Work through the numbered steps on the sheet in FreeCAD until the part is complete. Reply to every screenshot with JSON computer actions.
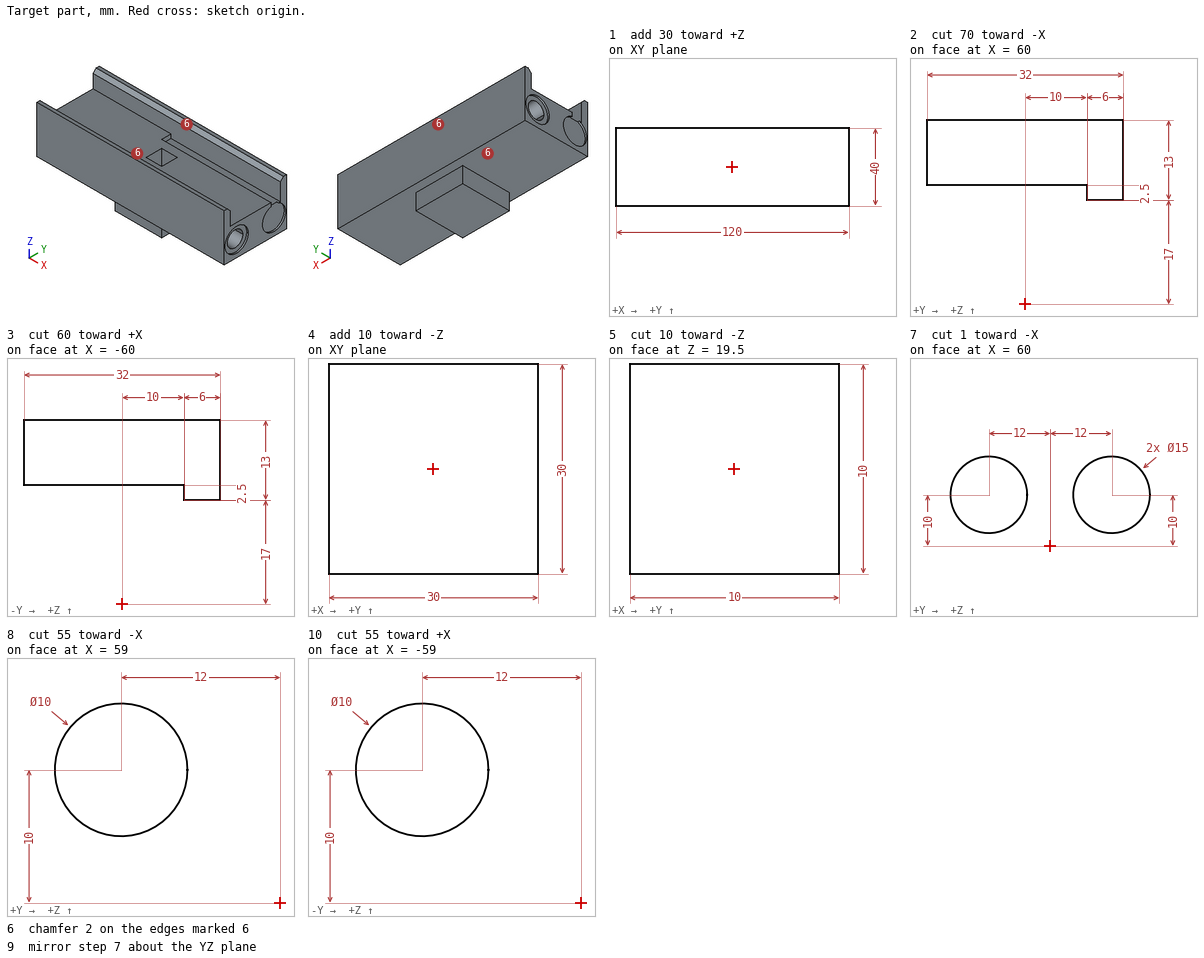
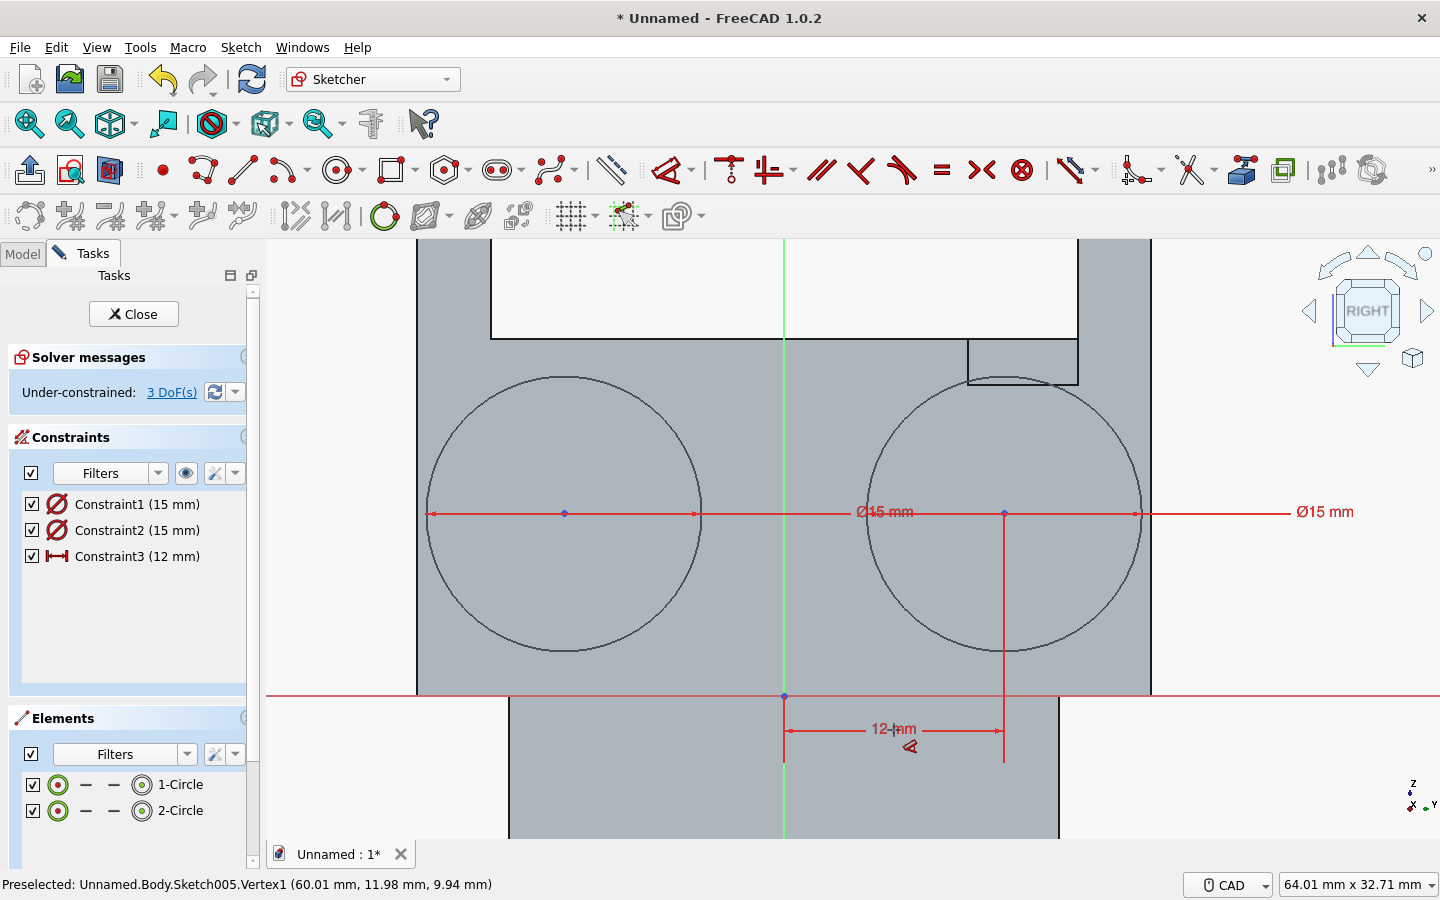
{"action": "left_click", "coordinate": [1004, 514]}
{"action": "left_click", "coordinate": [1038, 605]}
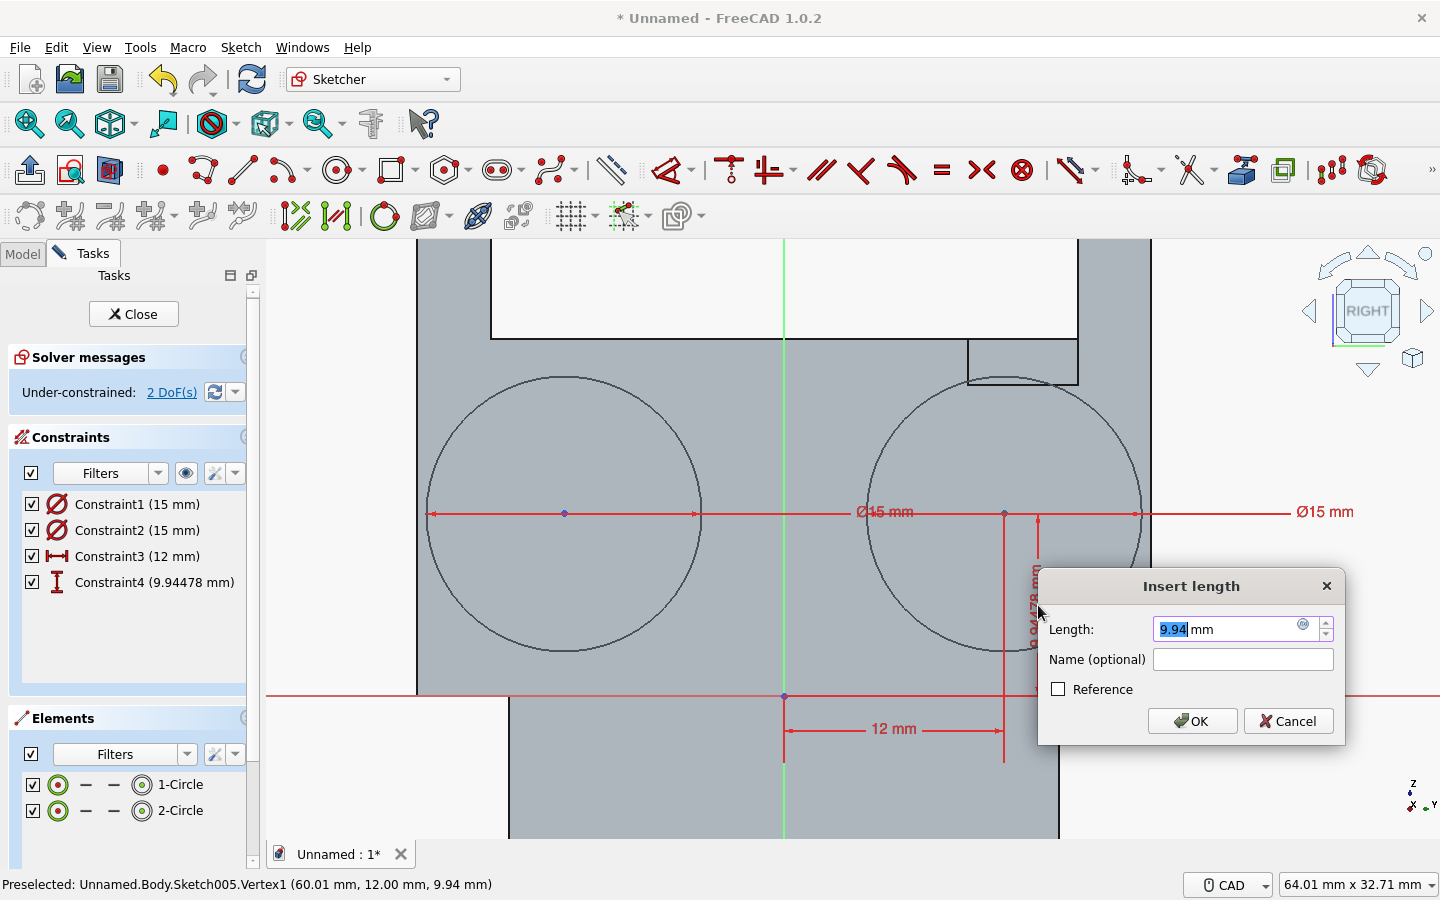
{"action": "type", "text": "10"}
{"action": "key", "text": "Return"}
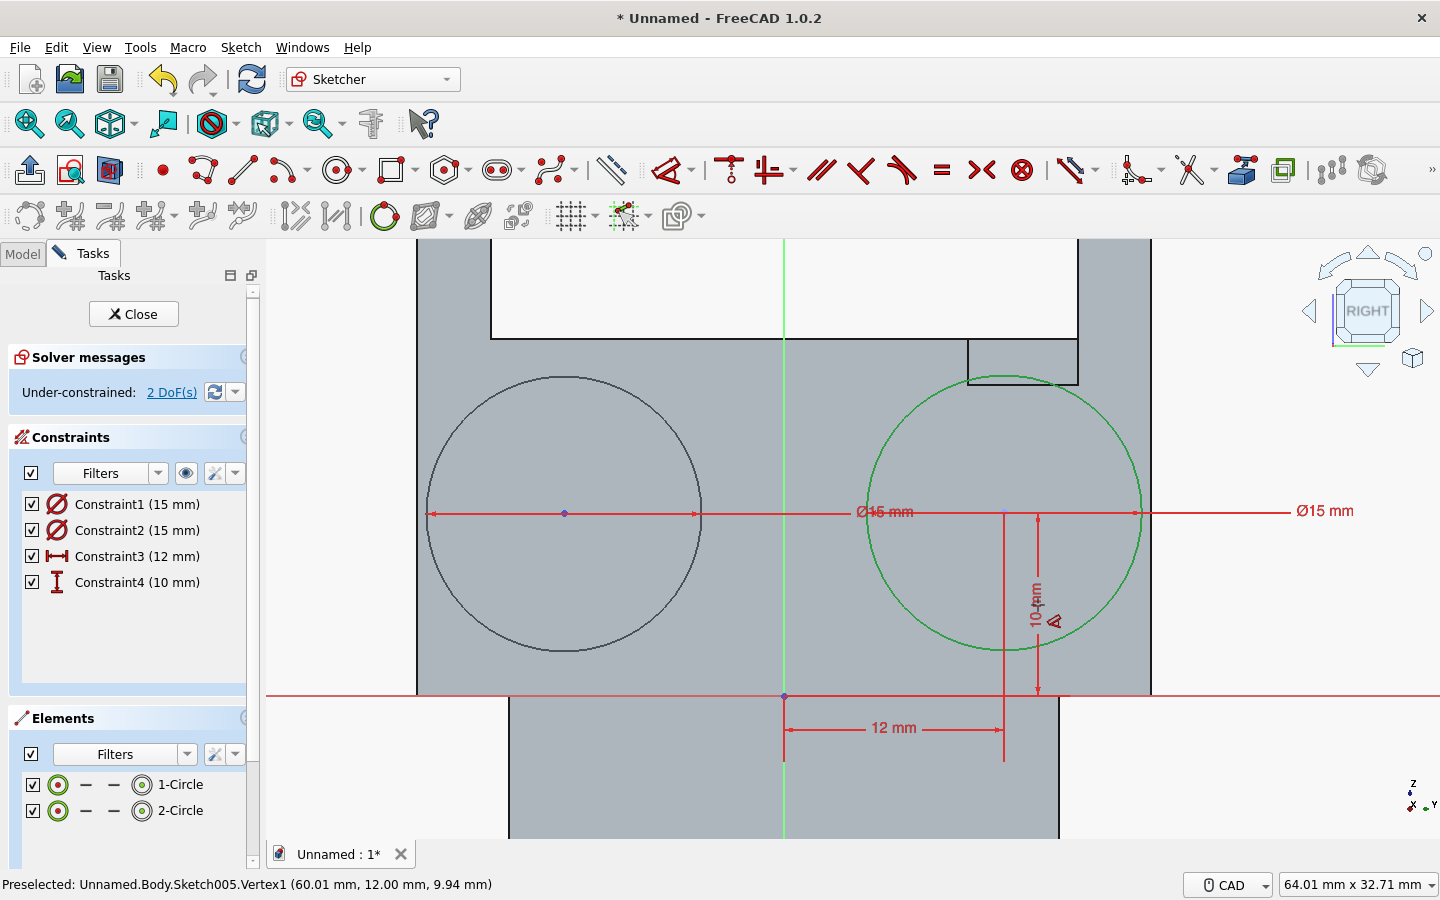
{"action": "left_click", "coordinate": [564, 514]}
{"action": "left_click", "coordinate": [674, 730]}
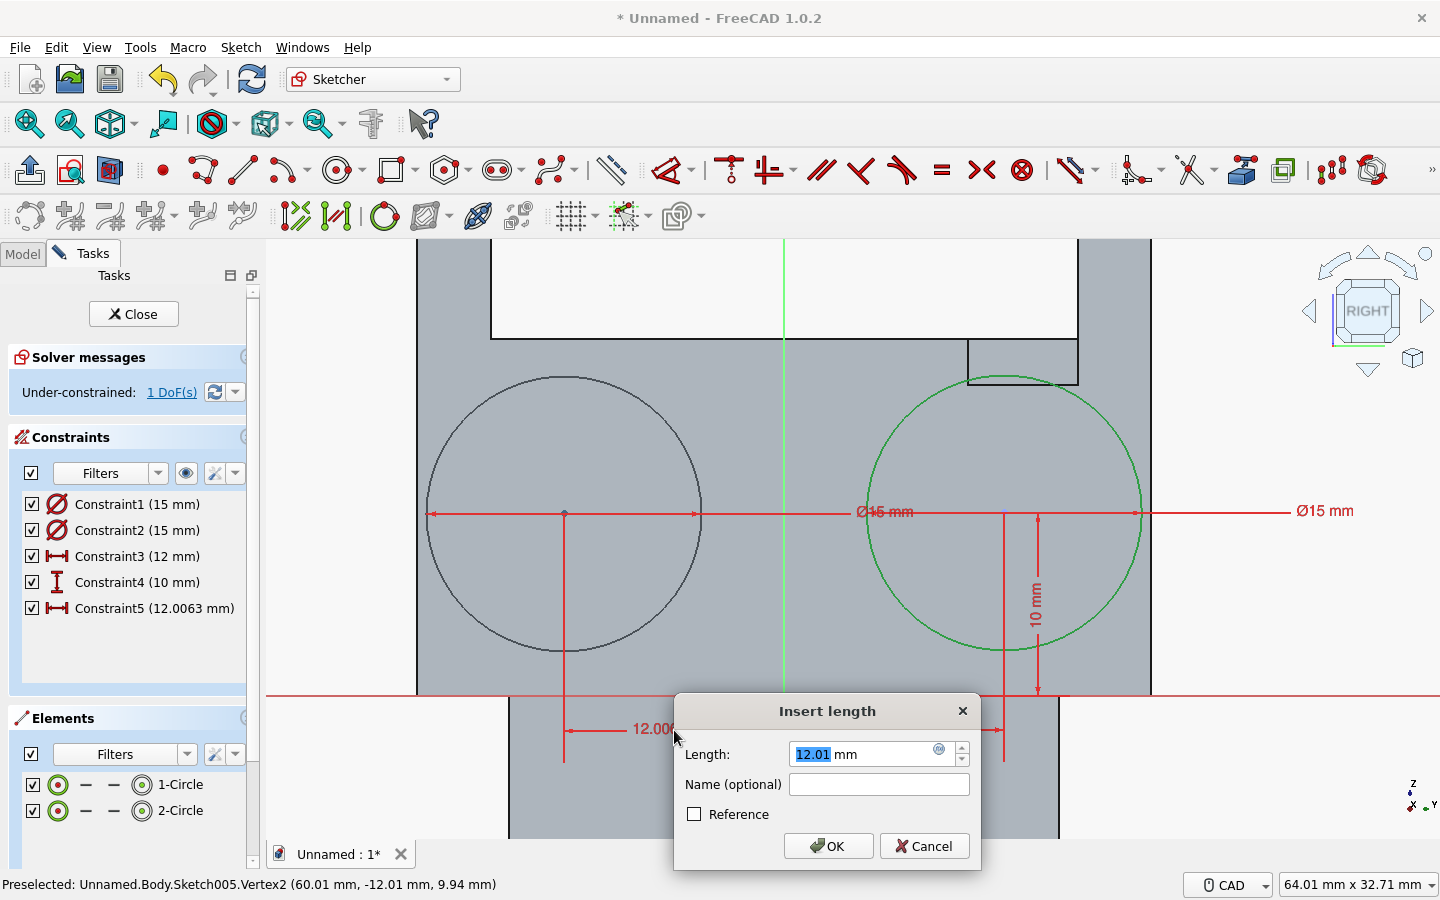
{"action": "type", "text": "12"}
{"action": "key", "text": "Return"}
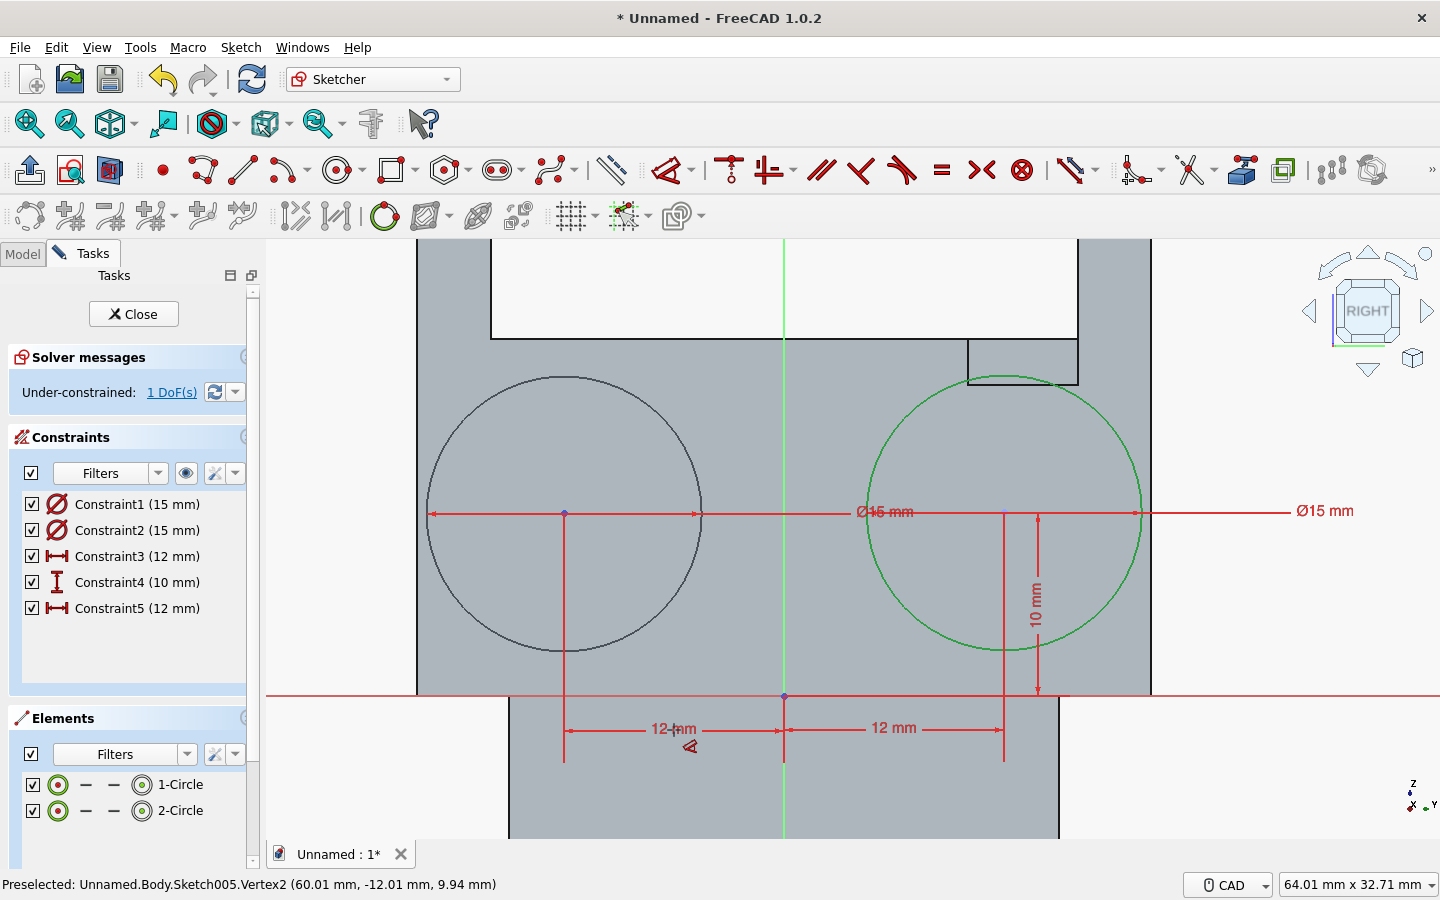
{"action": "left_click", "coordinate": [564, 514]}
{"action": "left_click", "coordinate": [530, 605]}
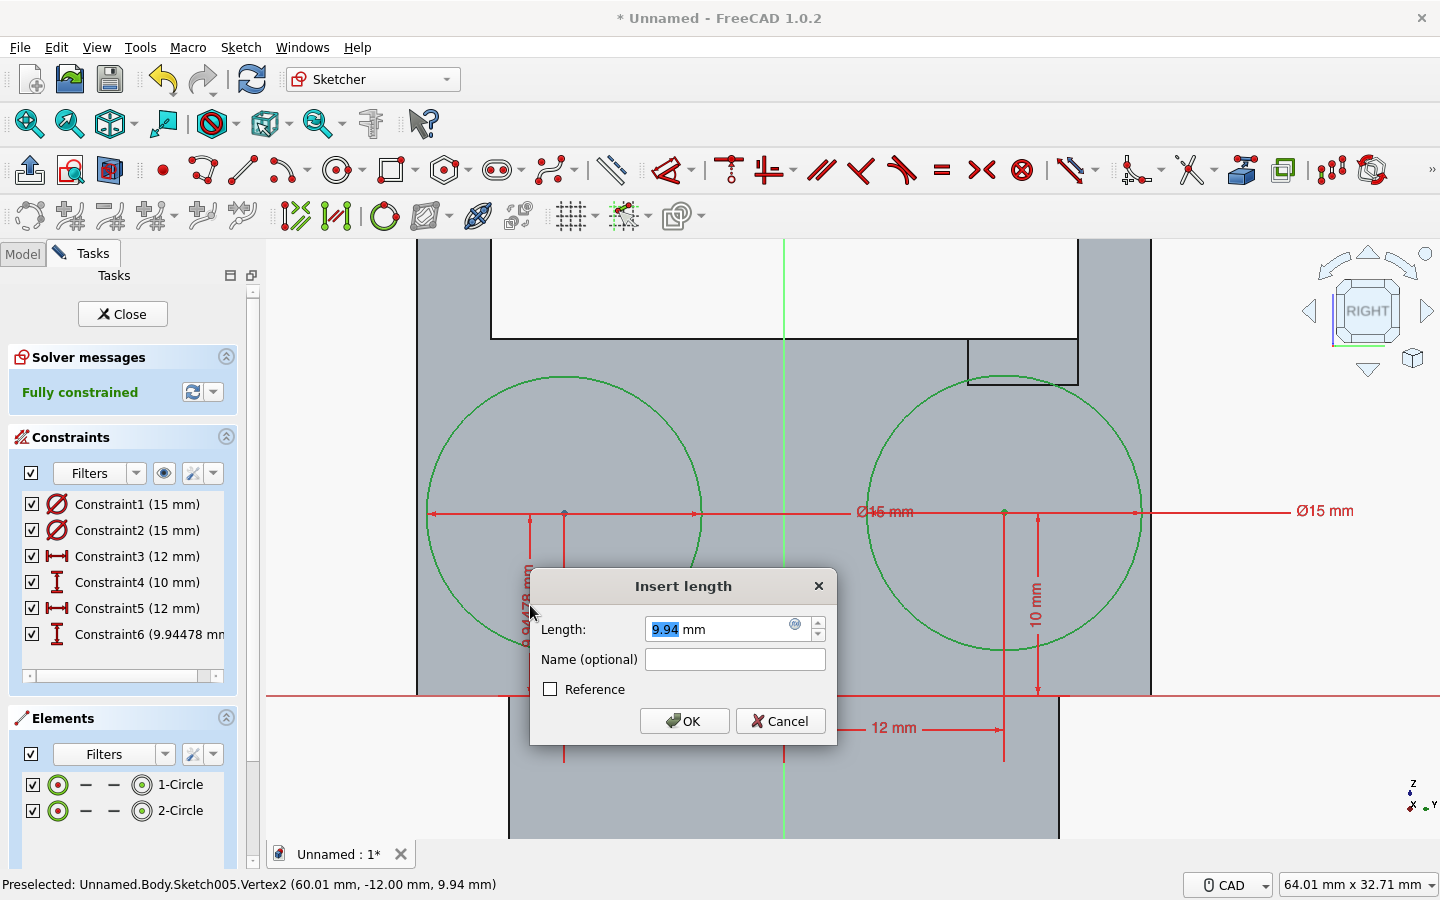
{"action": "type", "text": "10"}
{"action": "key", "text": "Return"}
{"action": "key", "text": "Escape"}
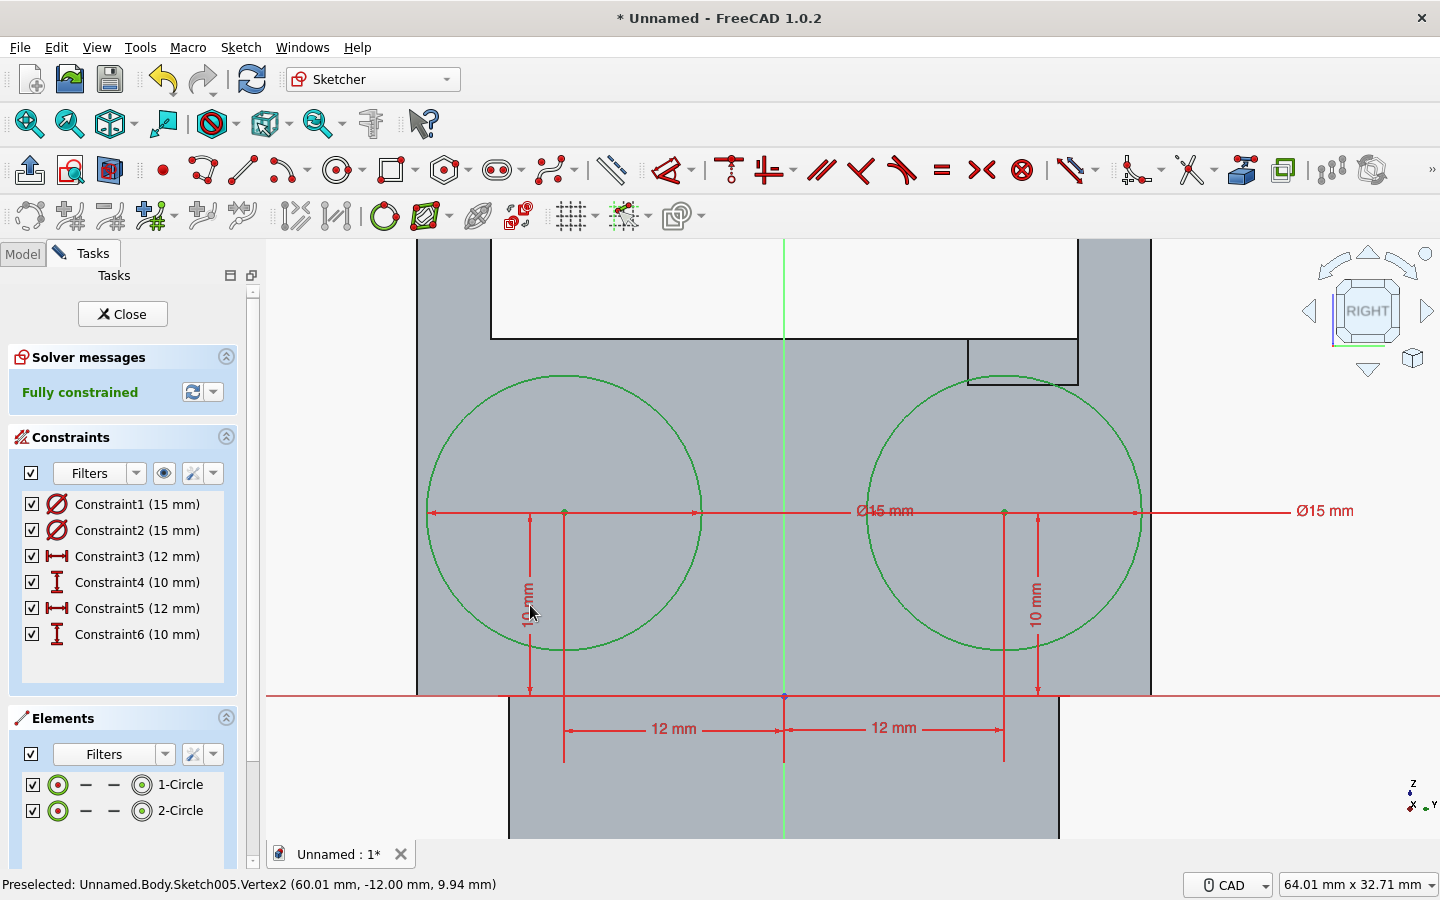
{"action": "left_click", "coordinate": [123, 314]}